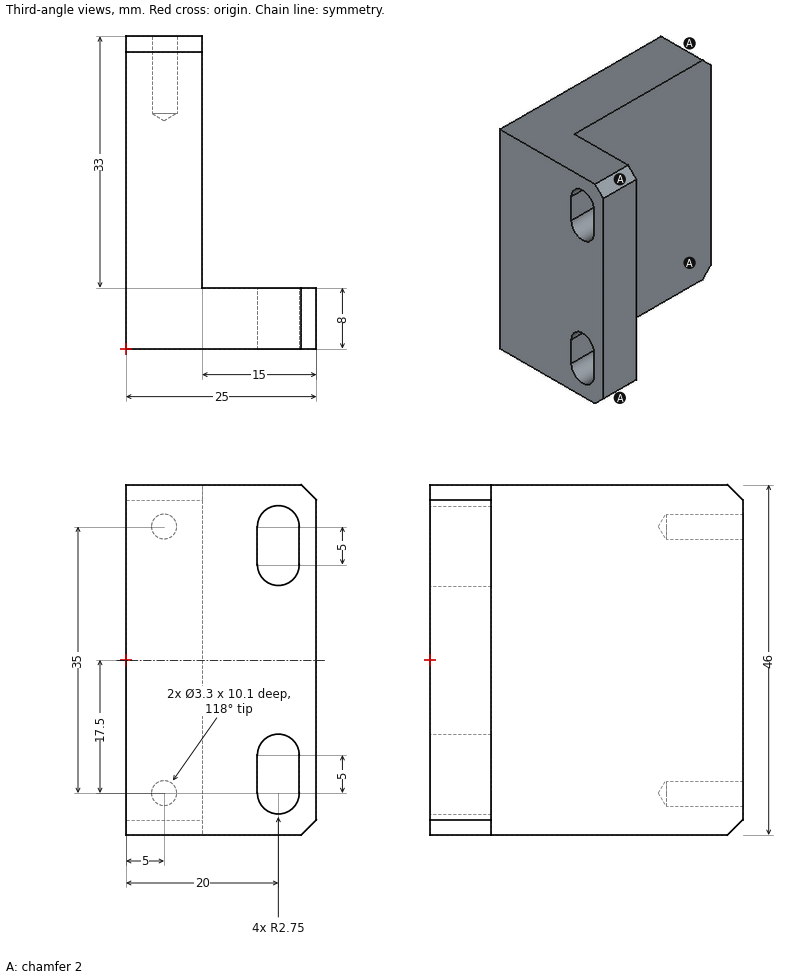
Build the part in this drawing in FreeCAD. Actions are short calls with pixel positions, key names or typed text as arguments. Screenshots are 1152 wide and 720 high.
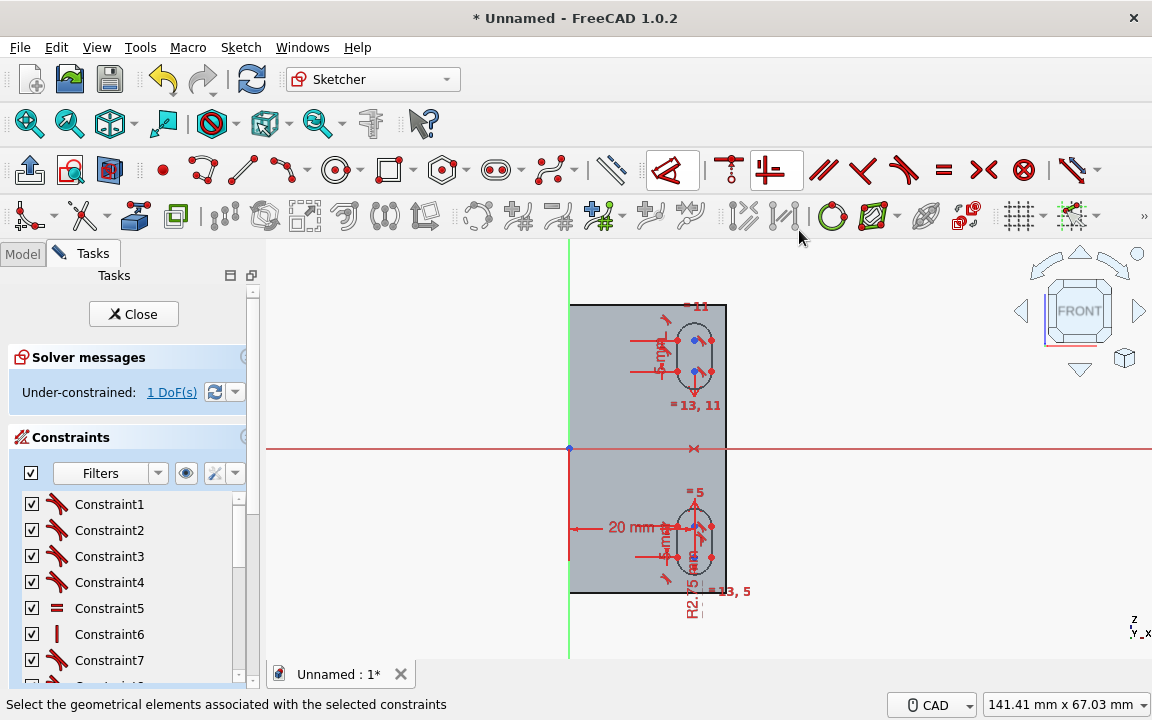
click(677, 557)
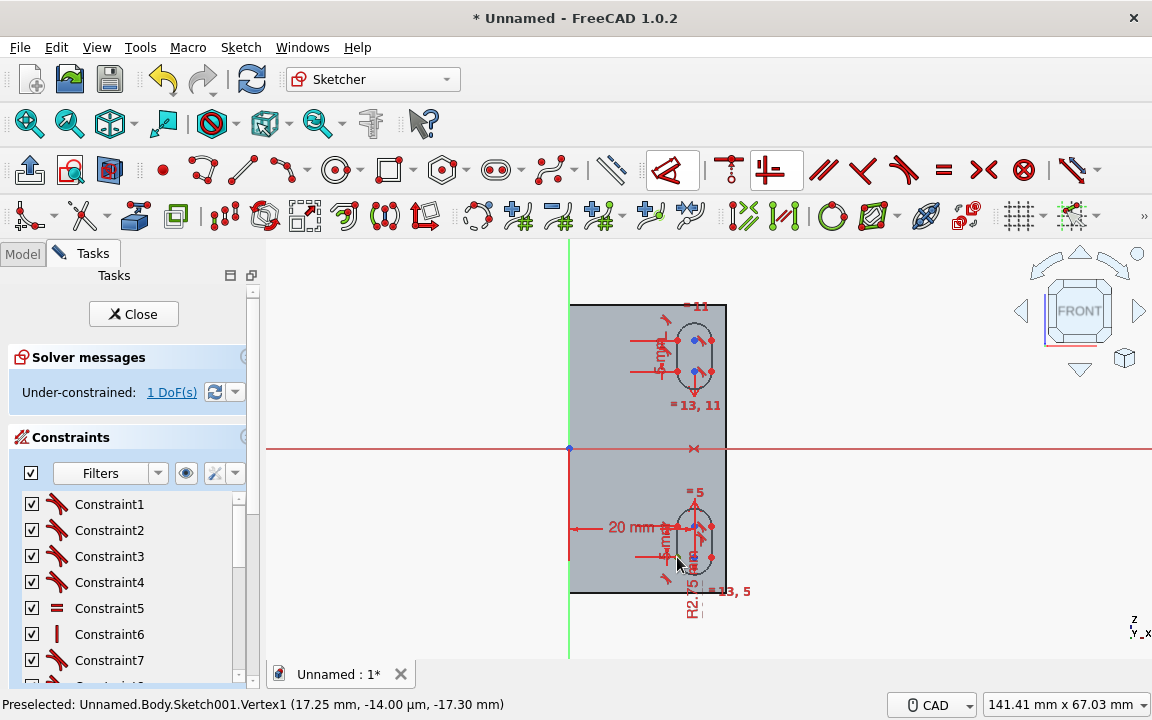
click(694, 170)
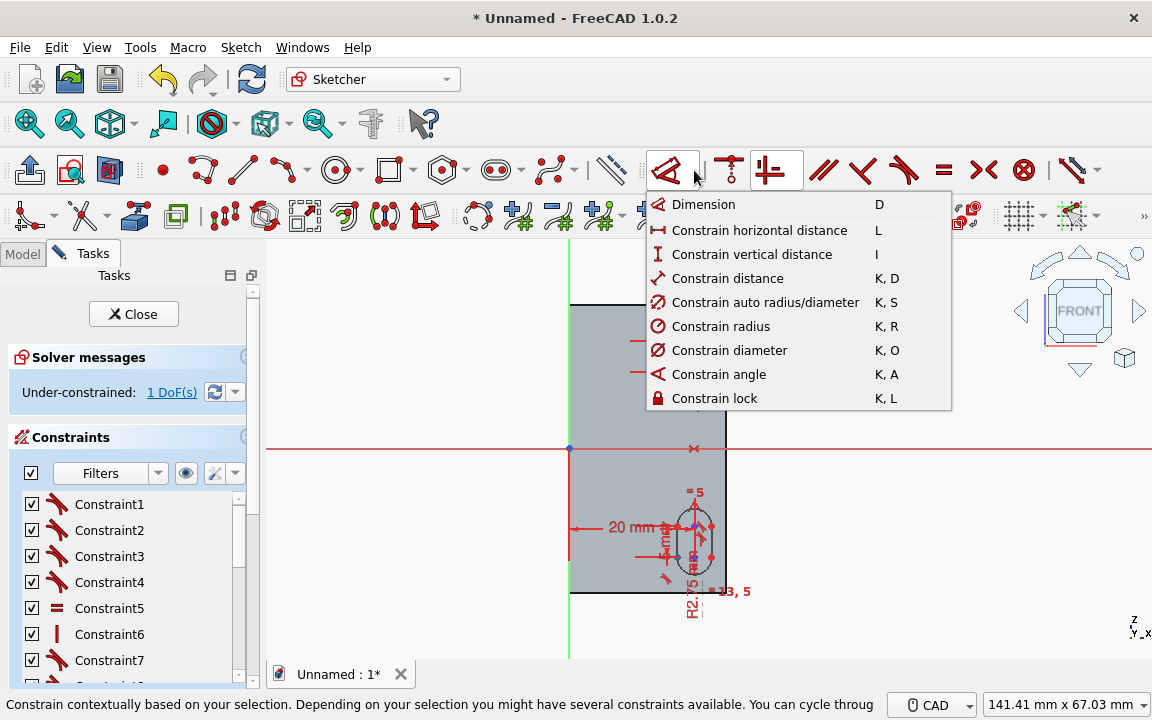
click(799, 254)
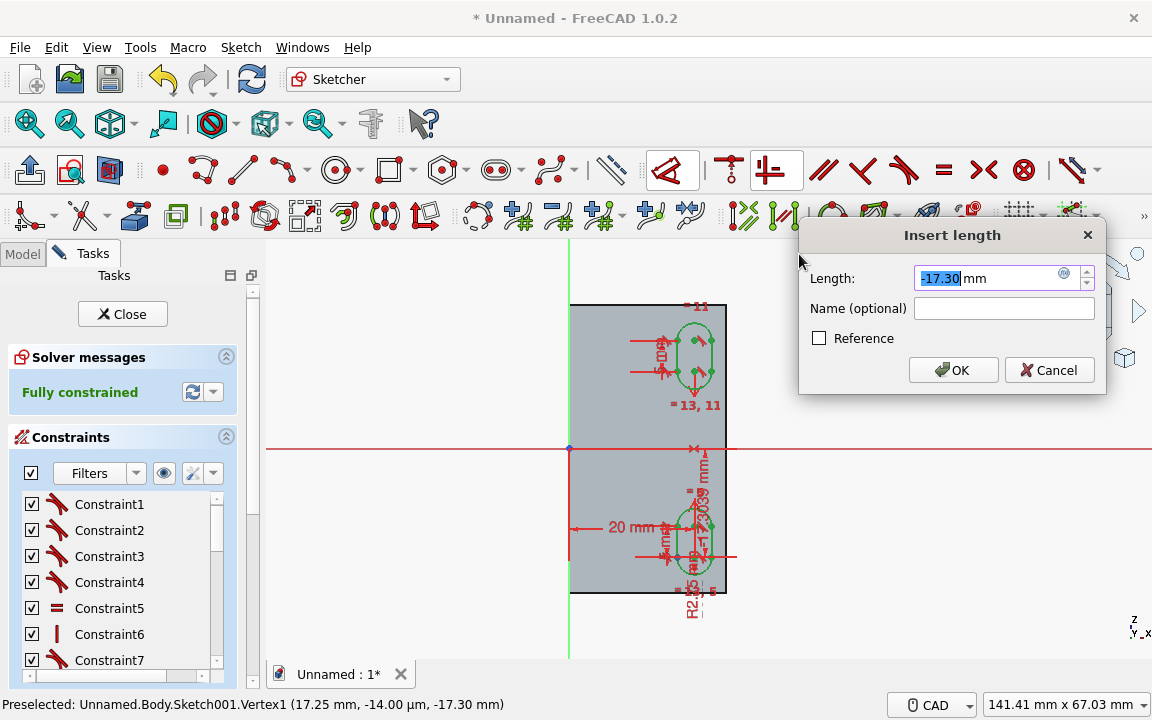
text(-17.5)
key(Return)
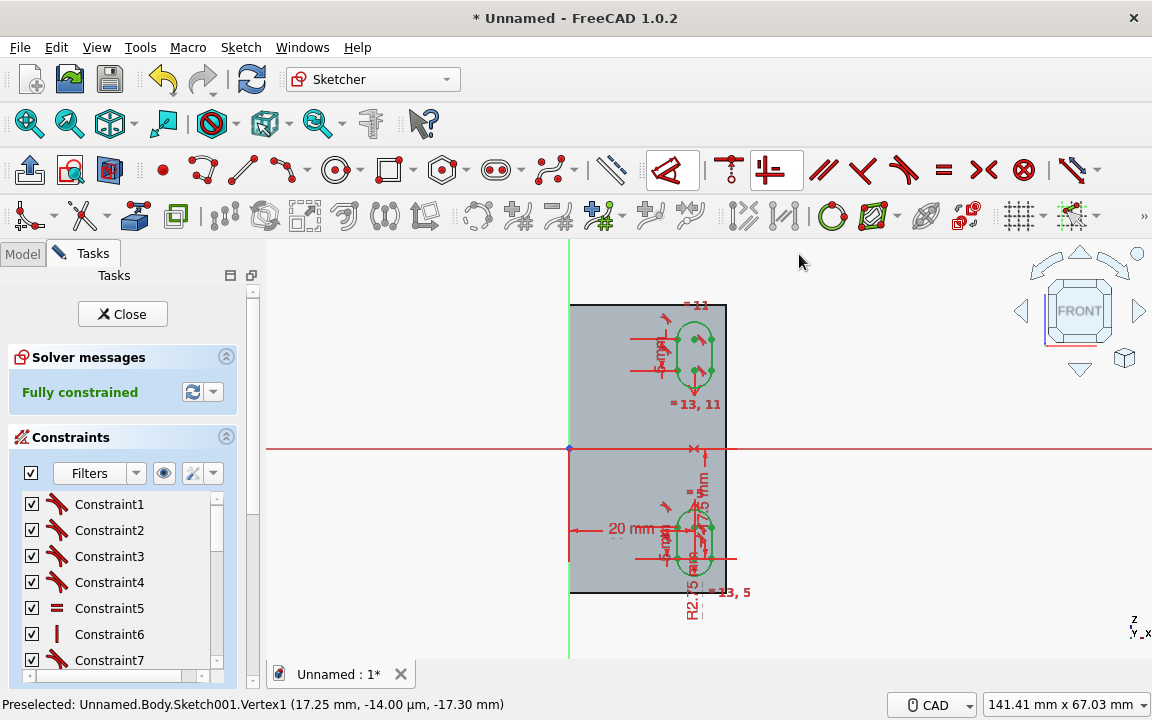
click(123, 314)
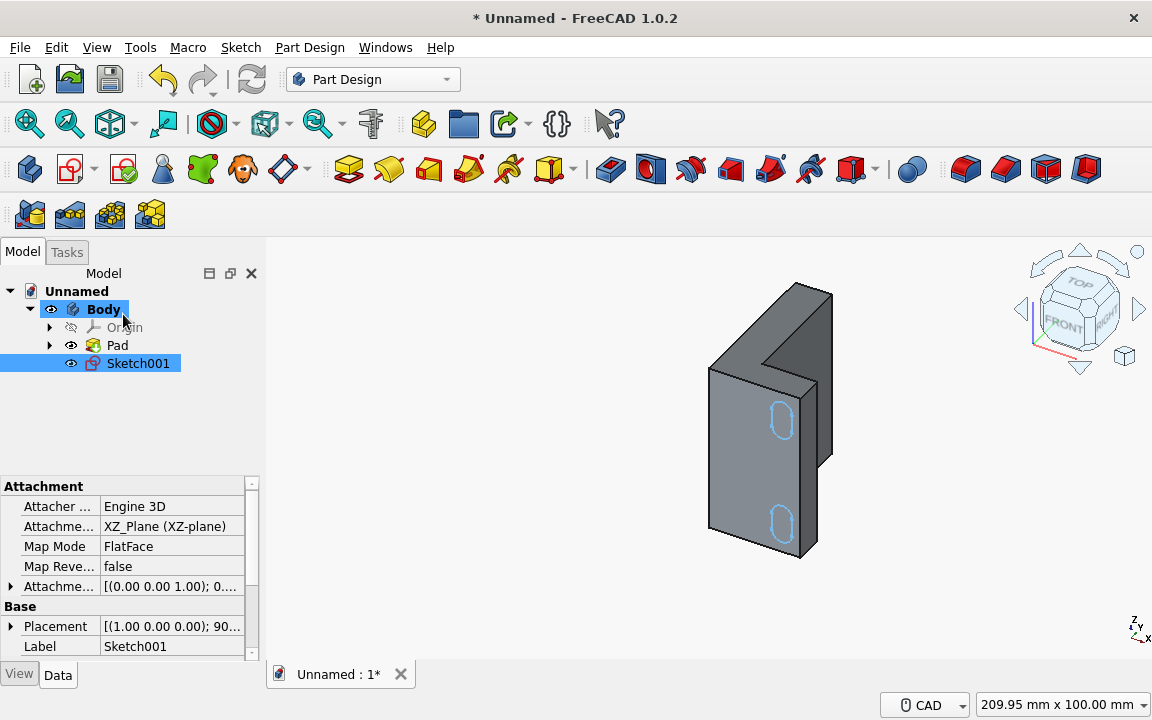
click(612, 170)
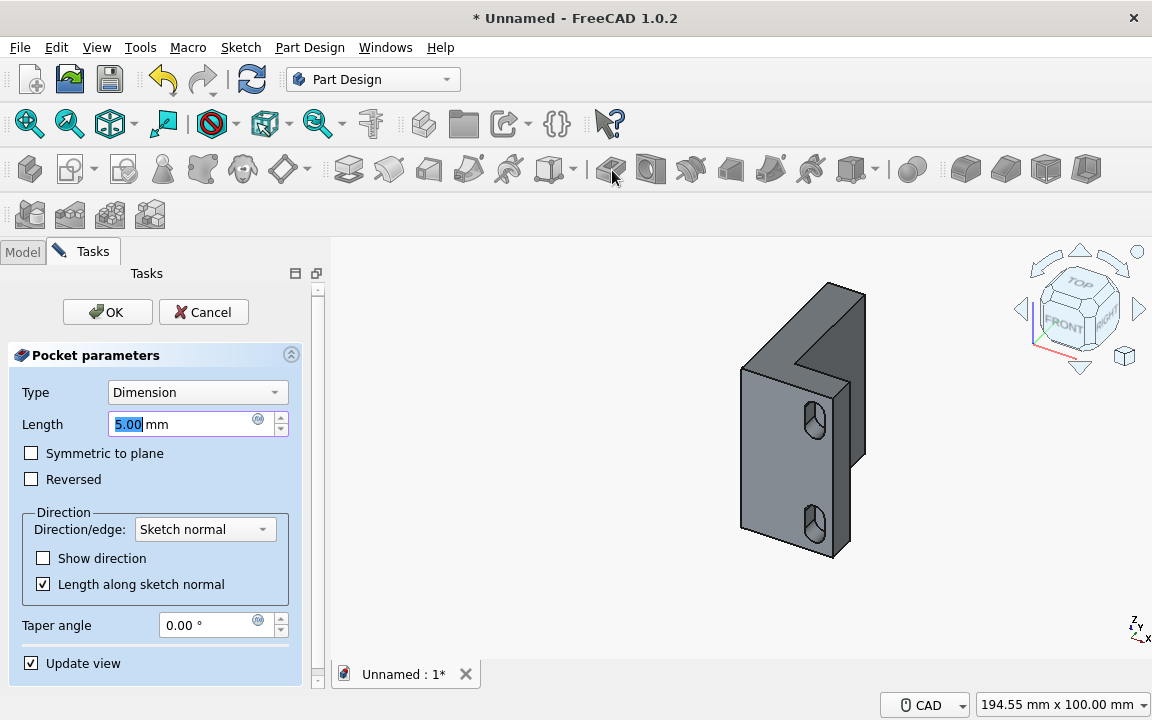
click(198, 392)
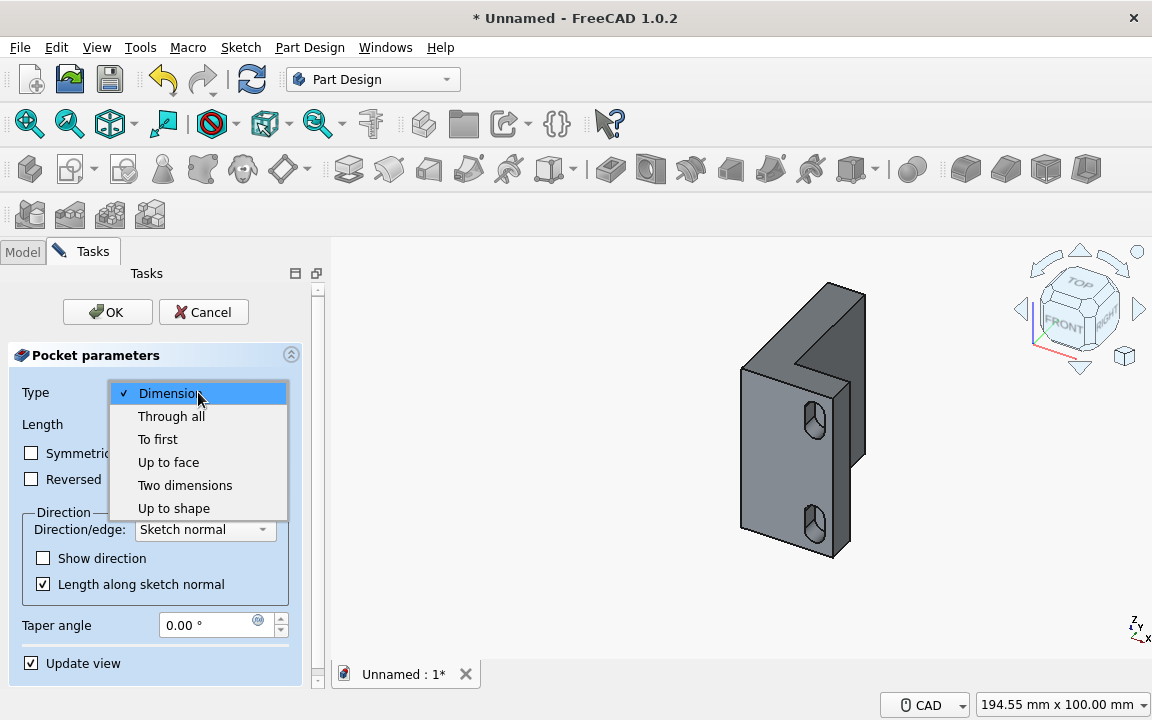
click(198, 416)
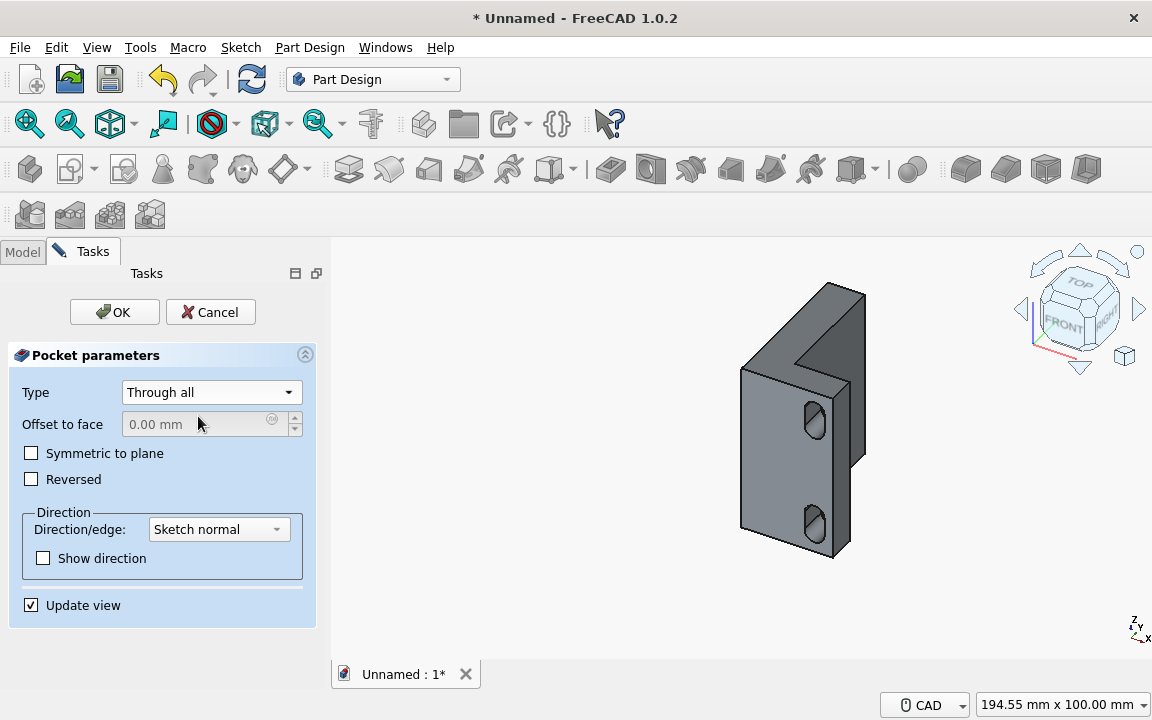
click(115, 312)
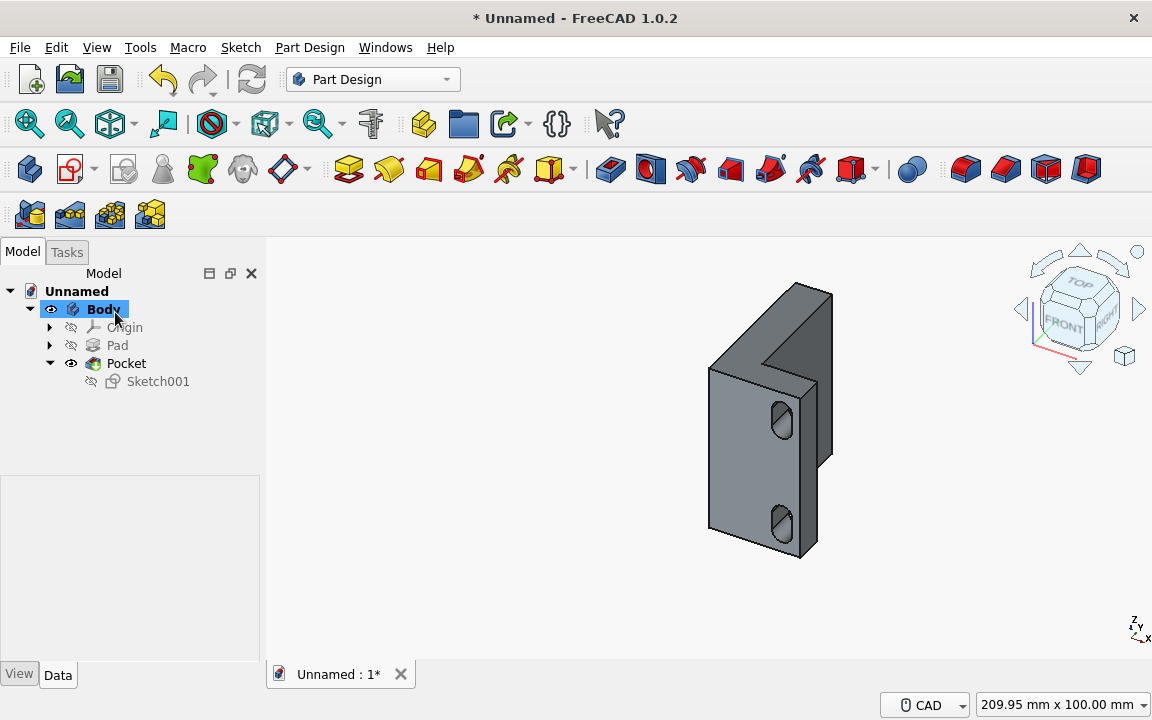
key(4)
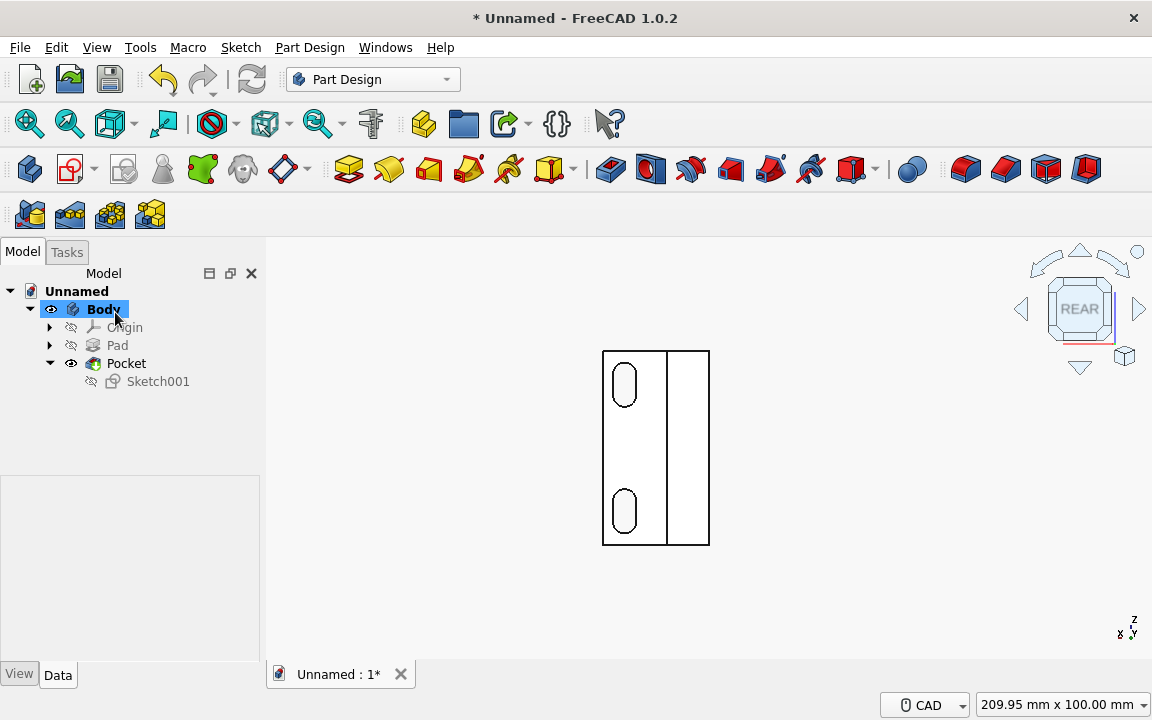
click(688, 392)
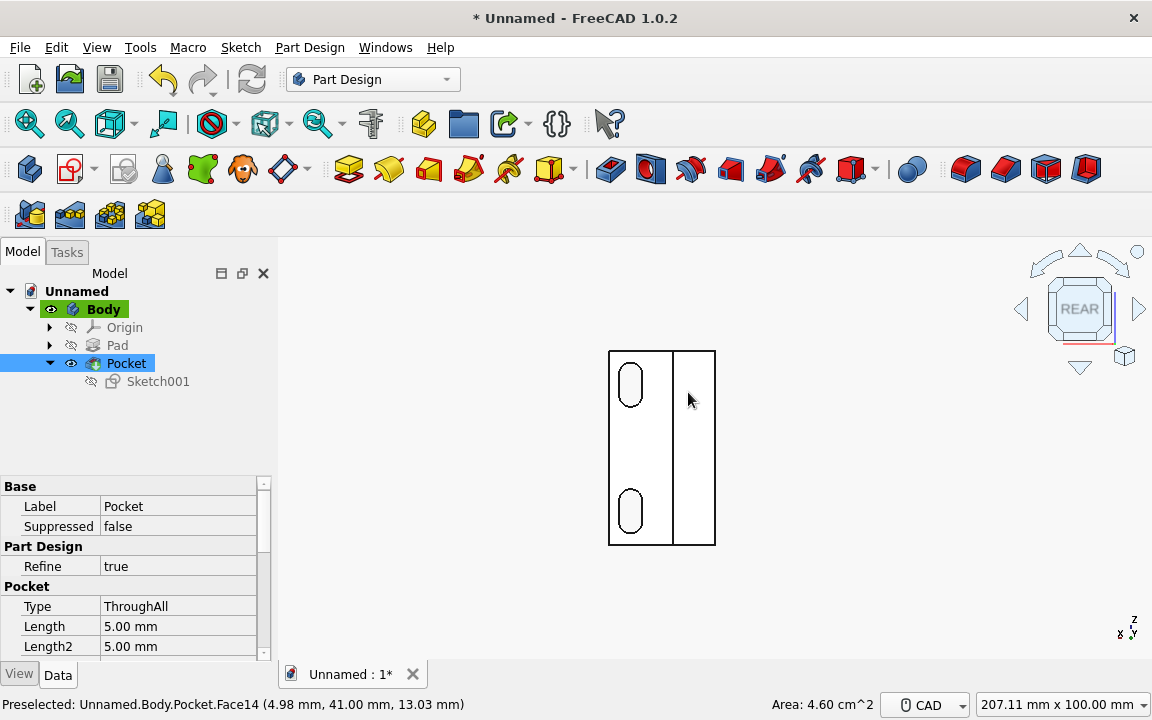
click(70, 170)